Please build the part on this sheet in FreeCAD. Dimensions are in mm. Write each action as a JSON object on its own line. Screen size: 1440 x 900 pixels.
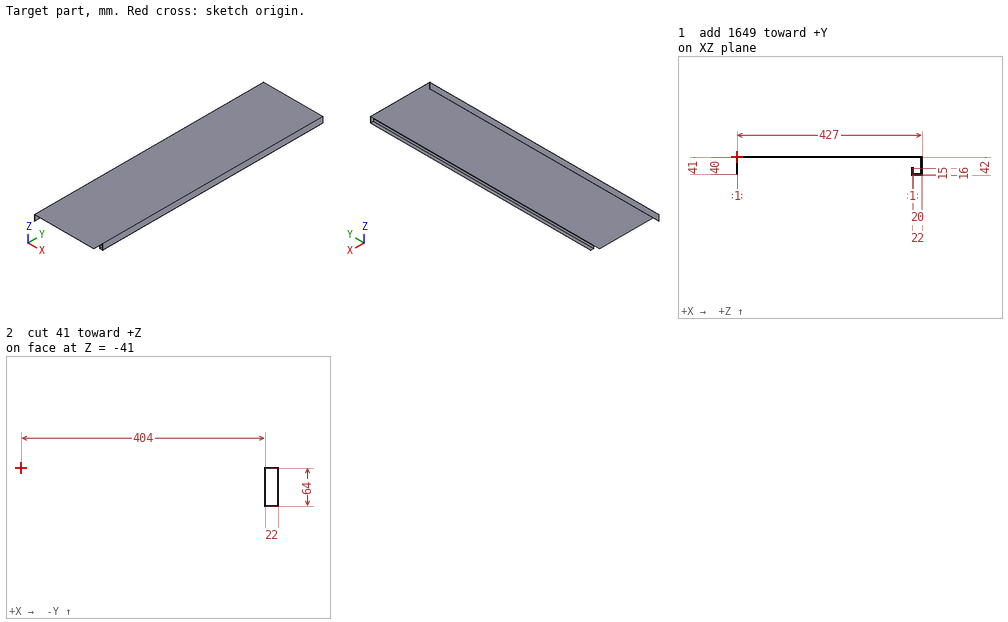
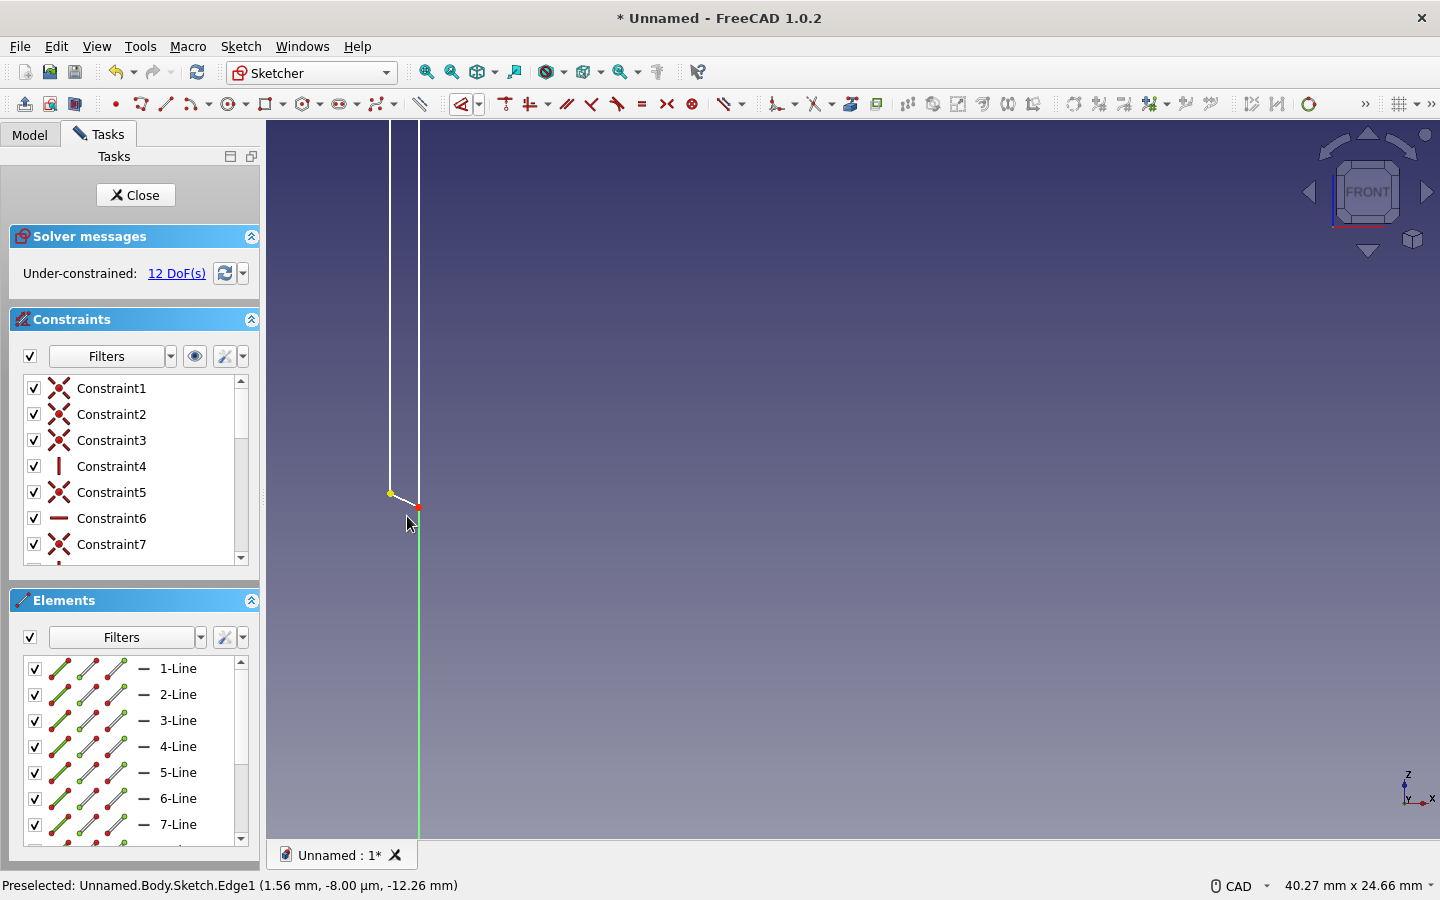
{"action": "left_click", "coordinate": [405, 501]}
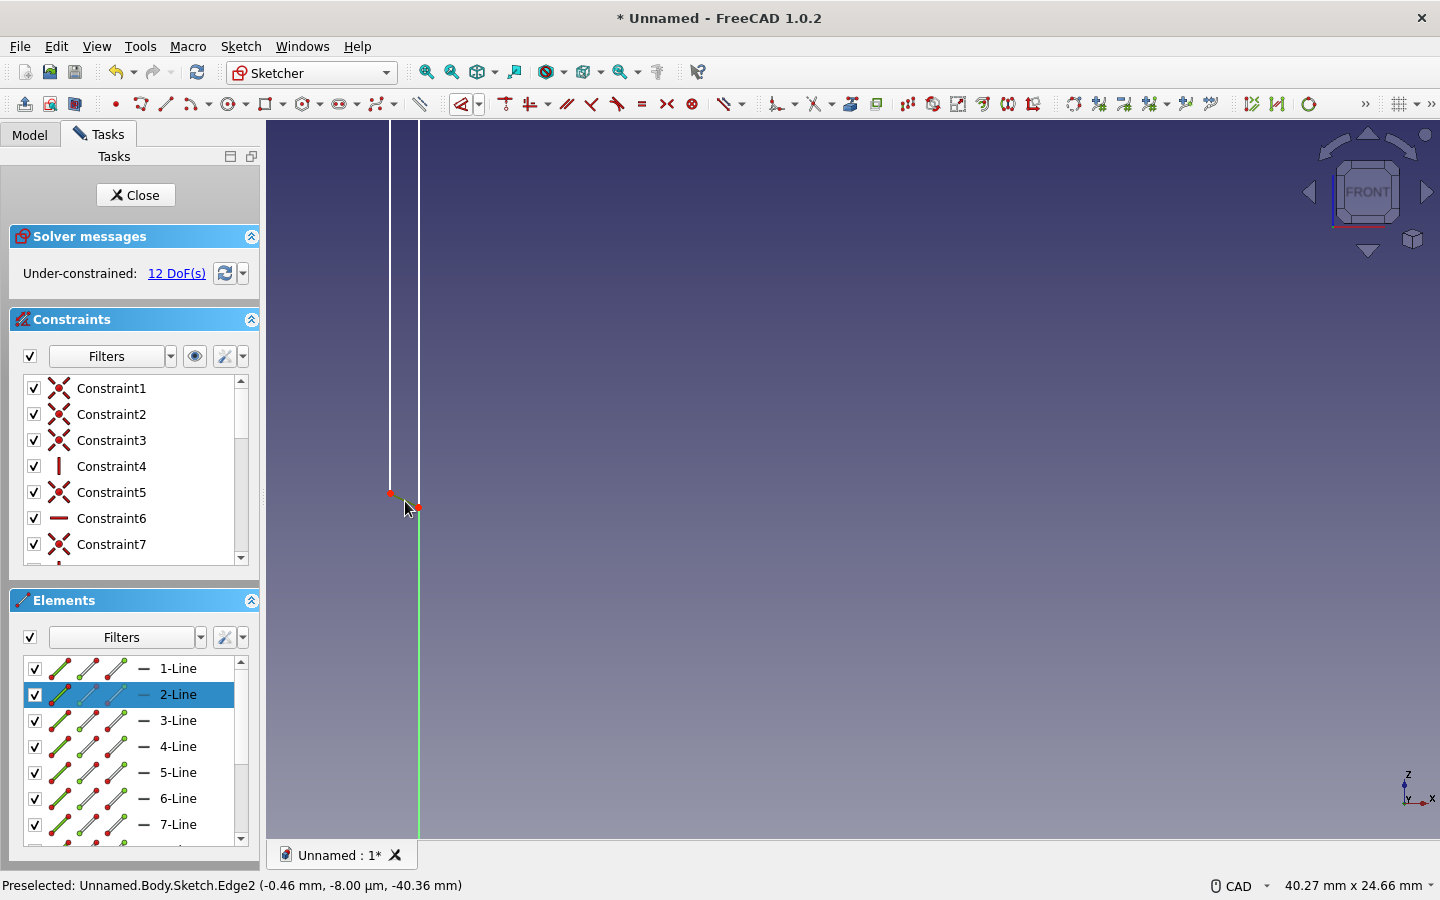
{"action": "left_click", "coordinate": [548, 104]}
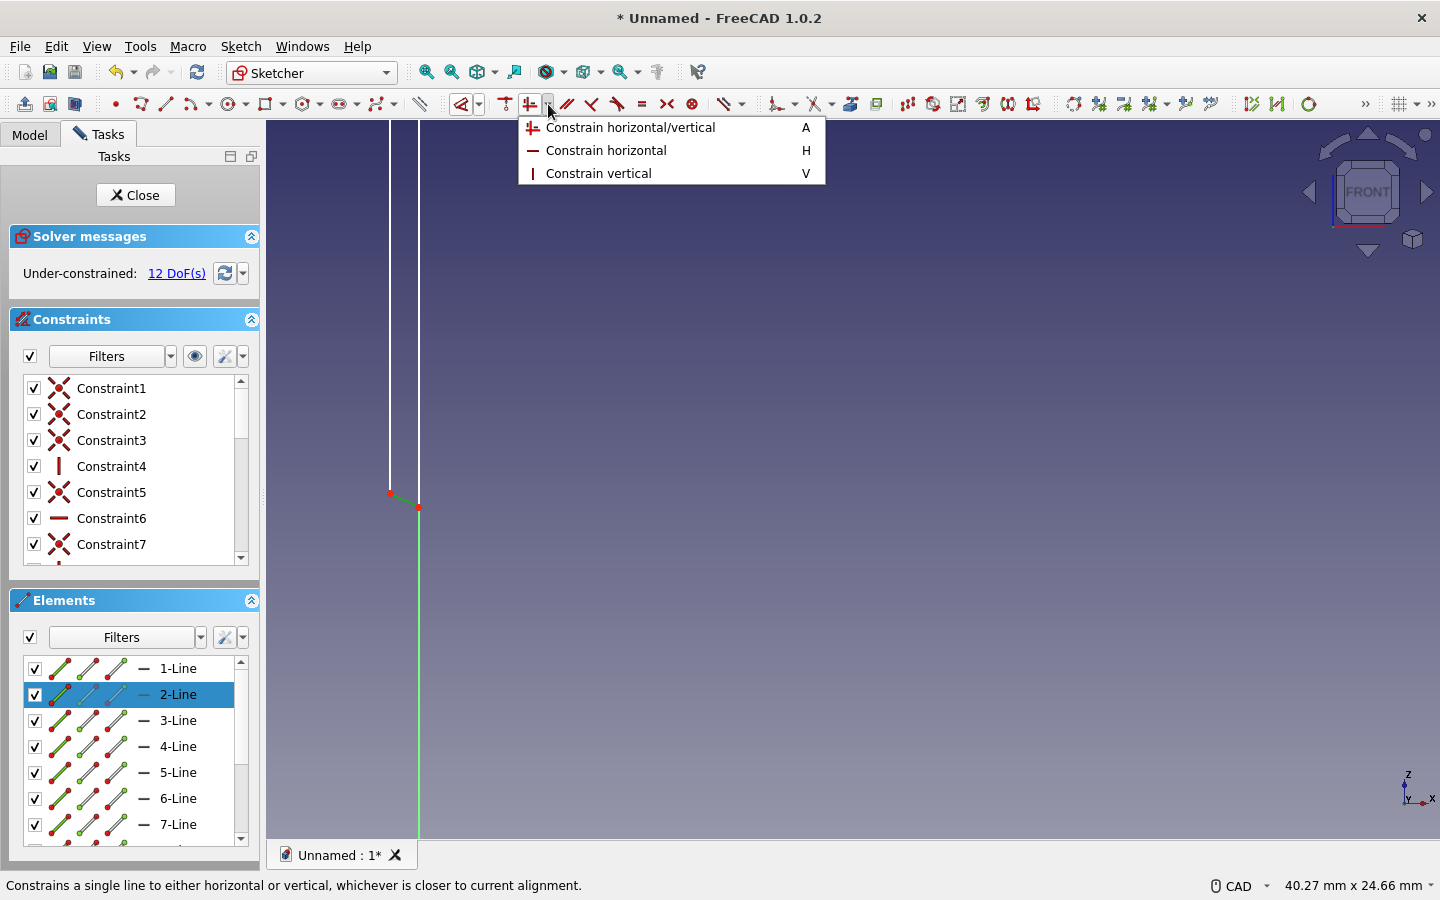
{"action": "left_click", "coordinate": [672, 150]}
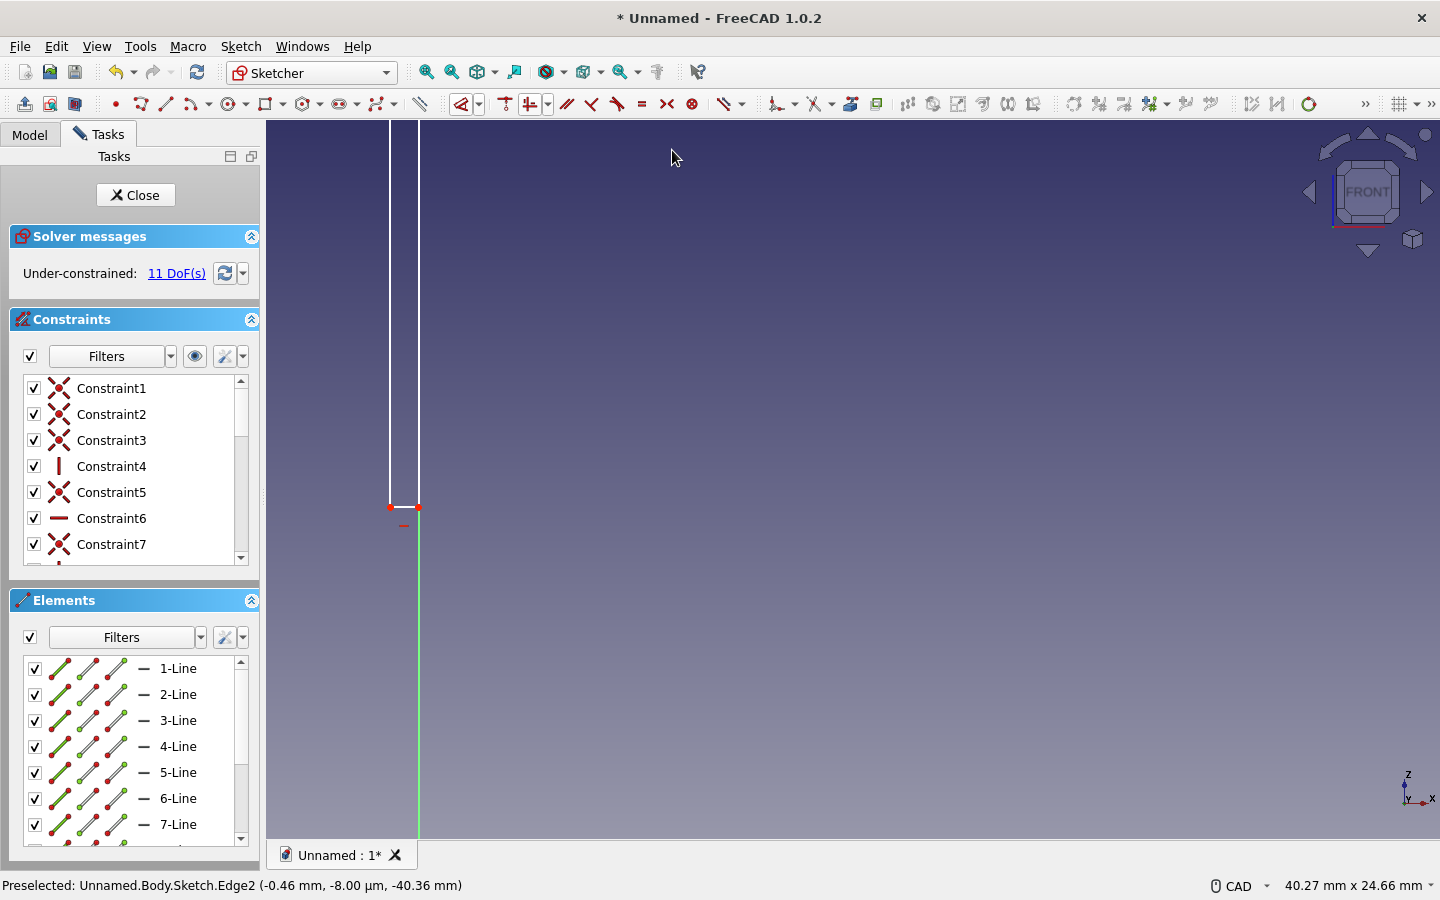
{"action": "scroll", "coordinate": [407, 517], "scroll_direction": "down", "scroll_amount": 14}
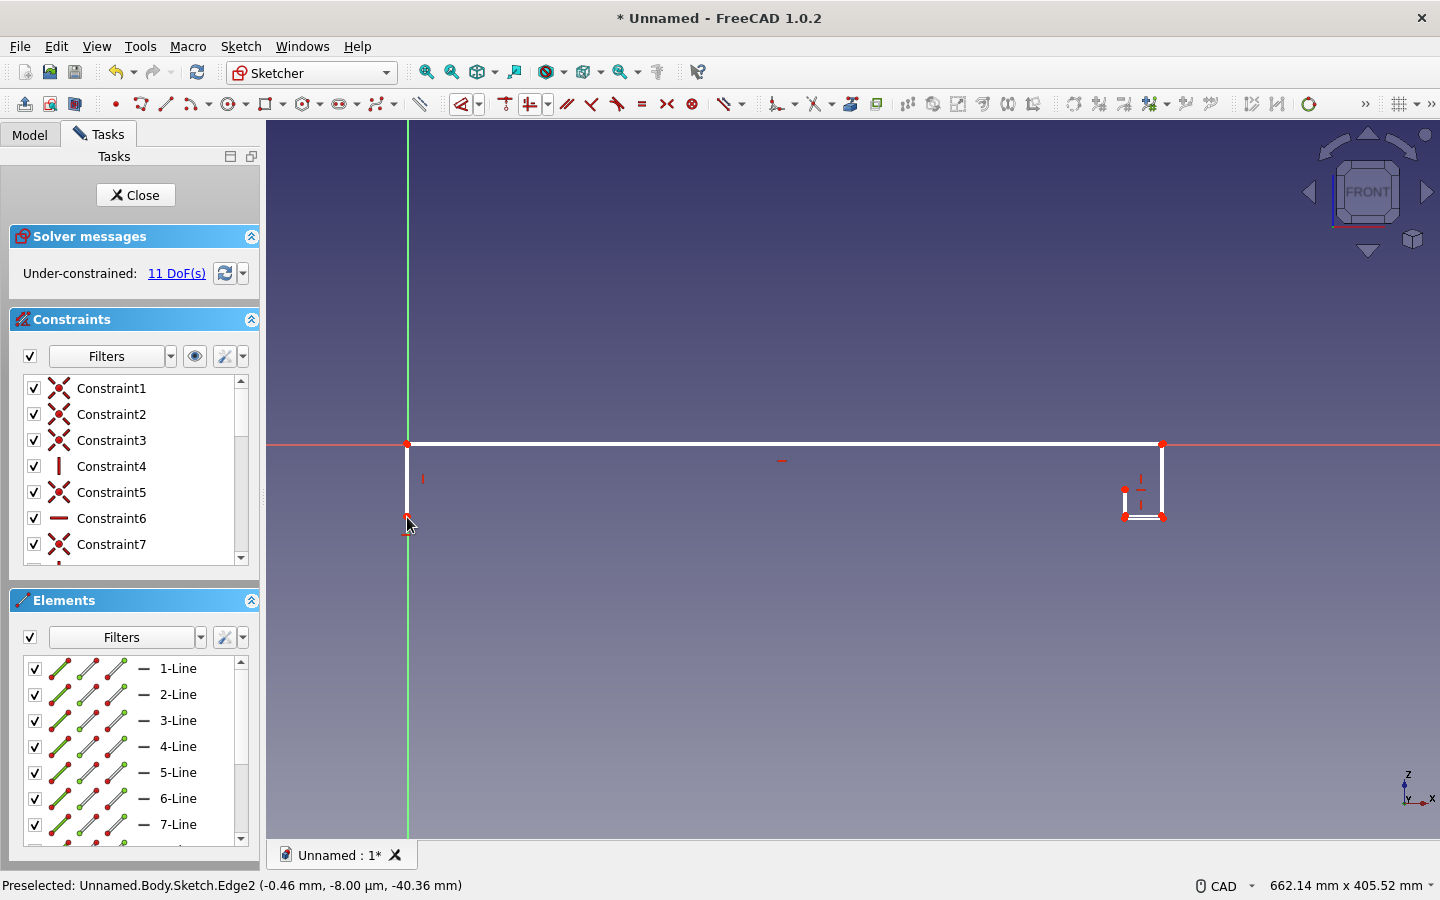
{"action": "scroll", "coordinate": [1125, 490], "scroll_direction": "up", "scroll_amount": 14}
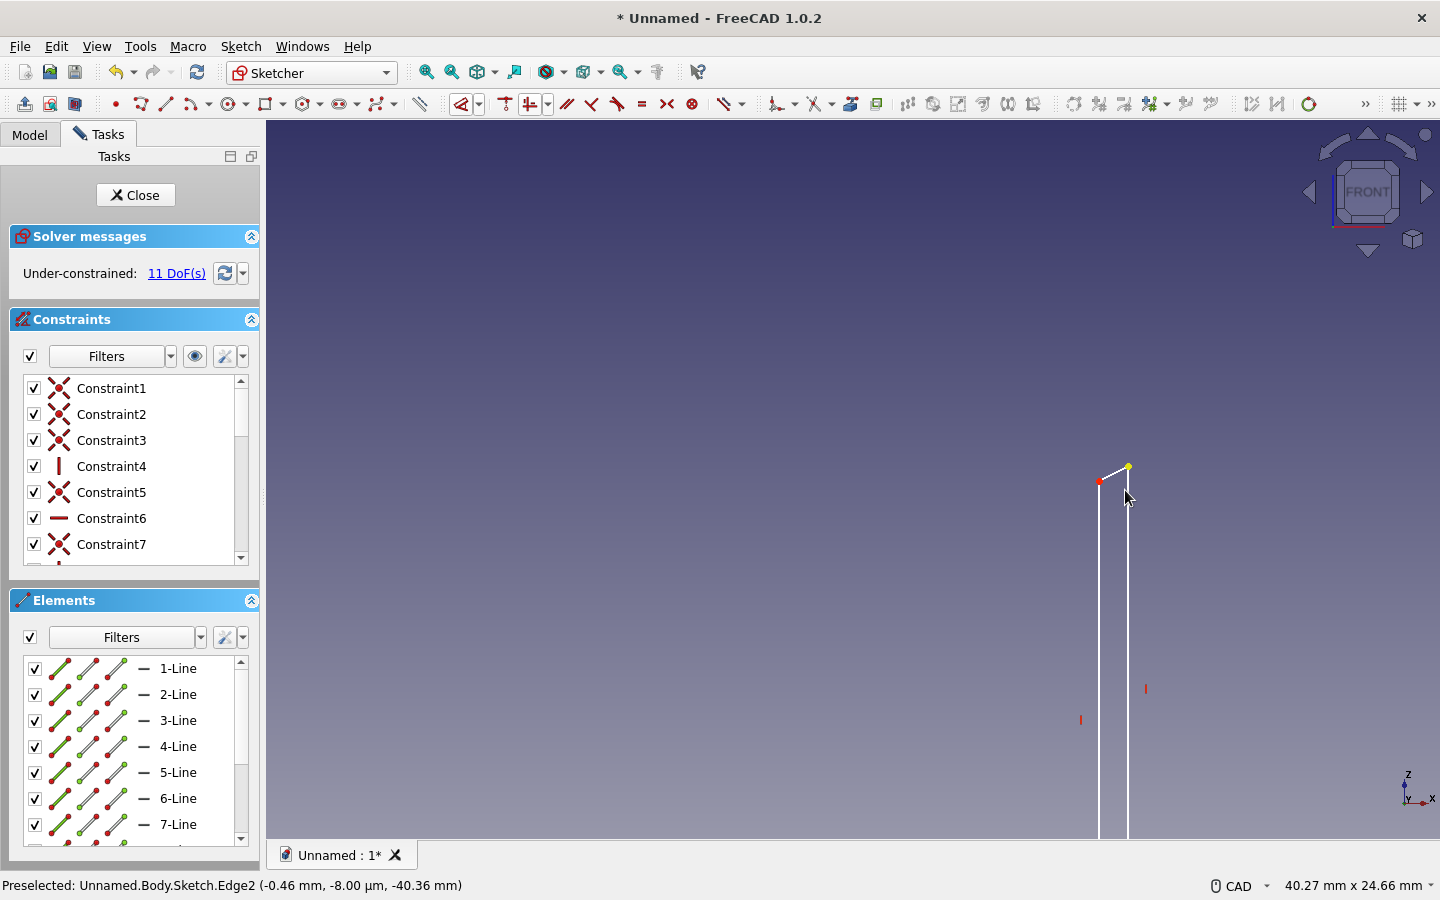
{"action": "left_click", "coordinate": [1108, 477]}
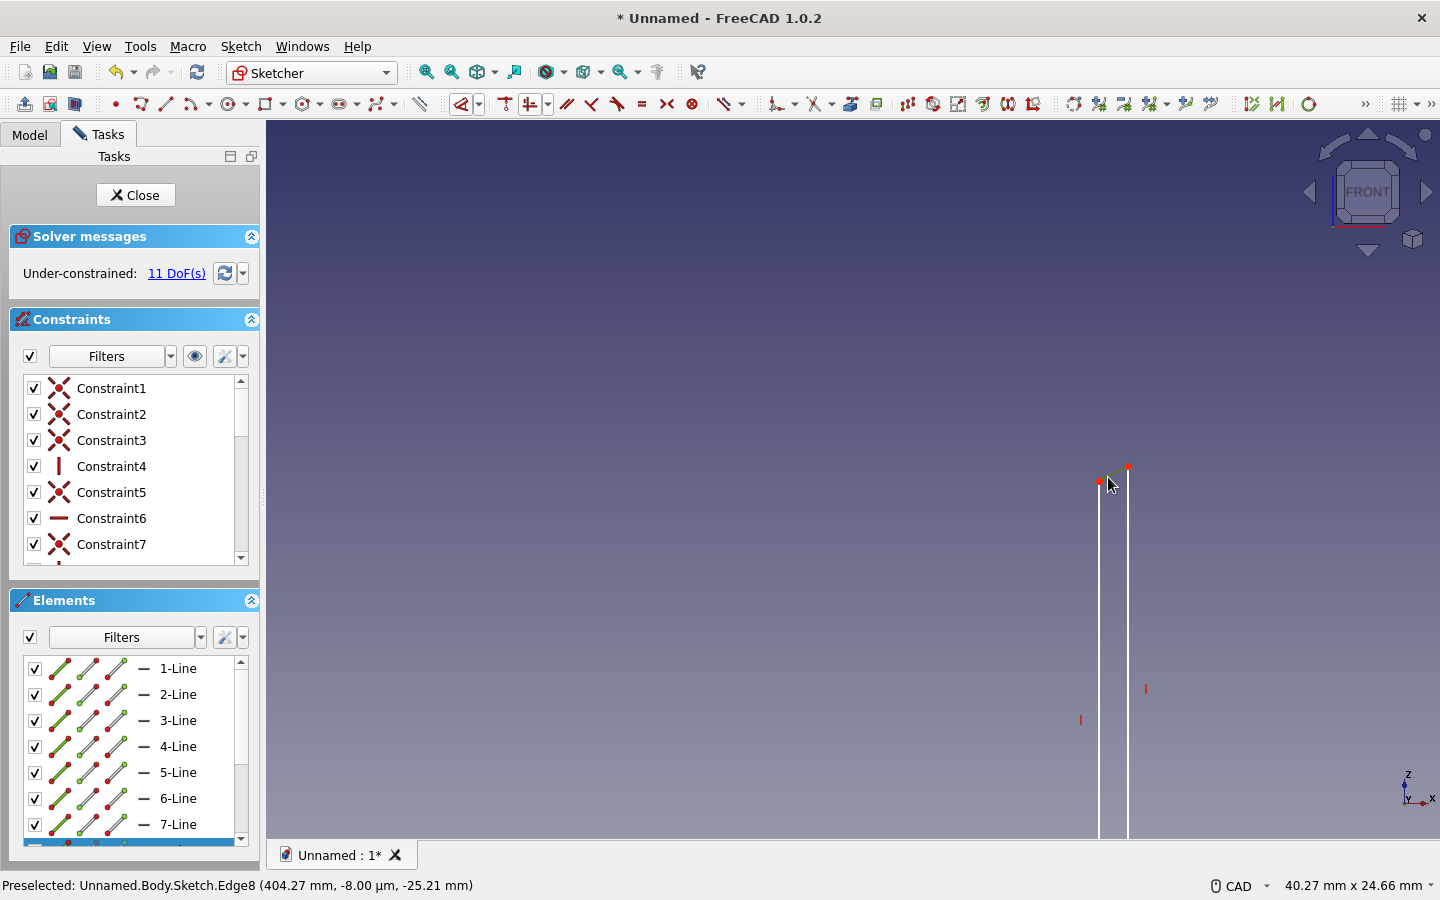
{"action": "key", "text": "h"}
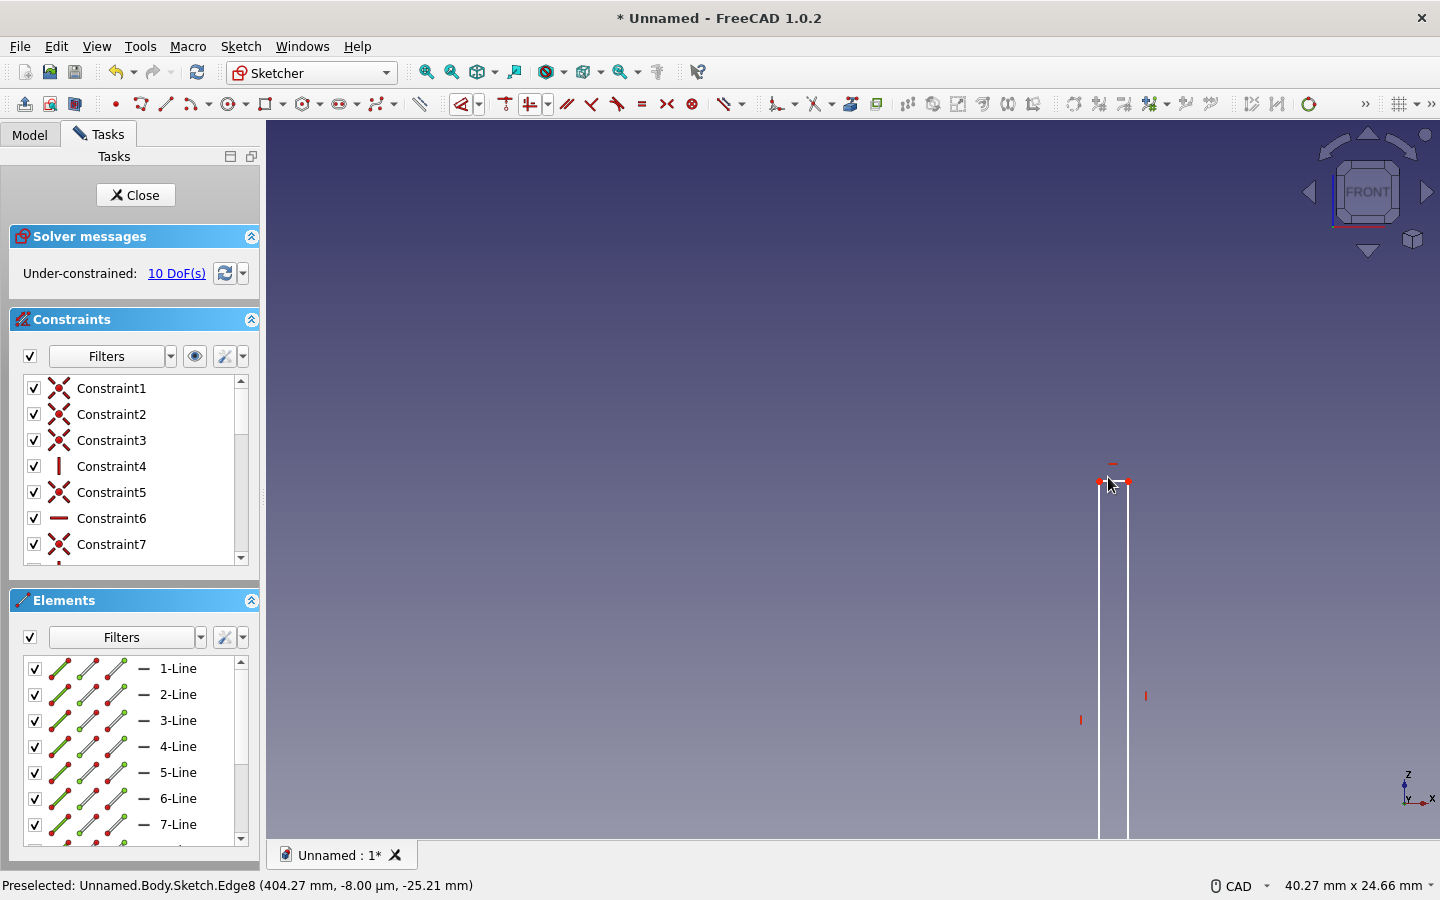
{"action": "left_click", "coordinate": [460, 104]}